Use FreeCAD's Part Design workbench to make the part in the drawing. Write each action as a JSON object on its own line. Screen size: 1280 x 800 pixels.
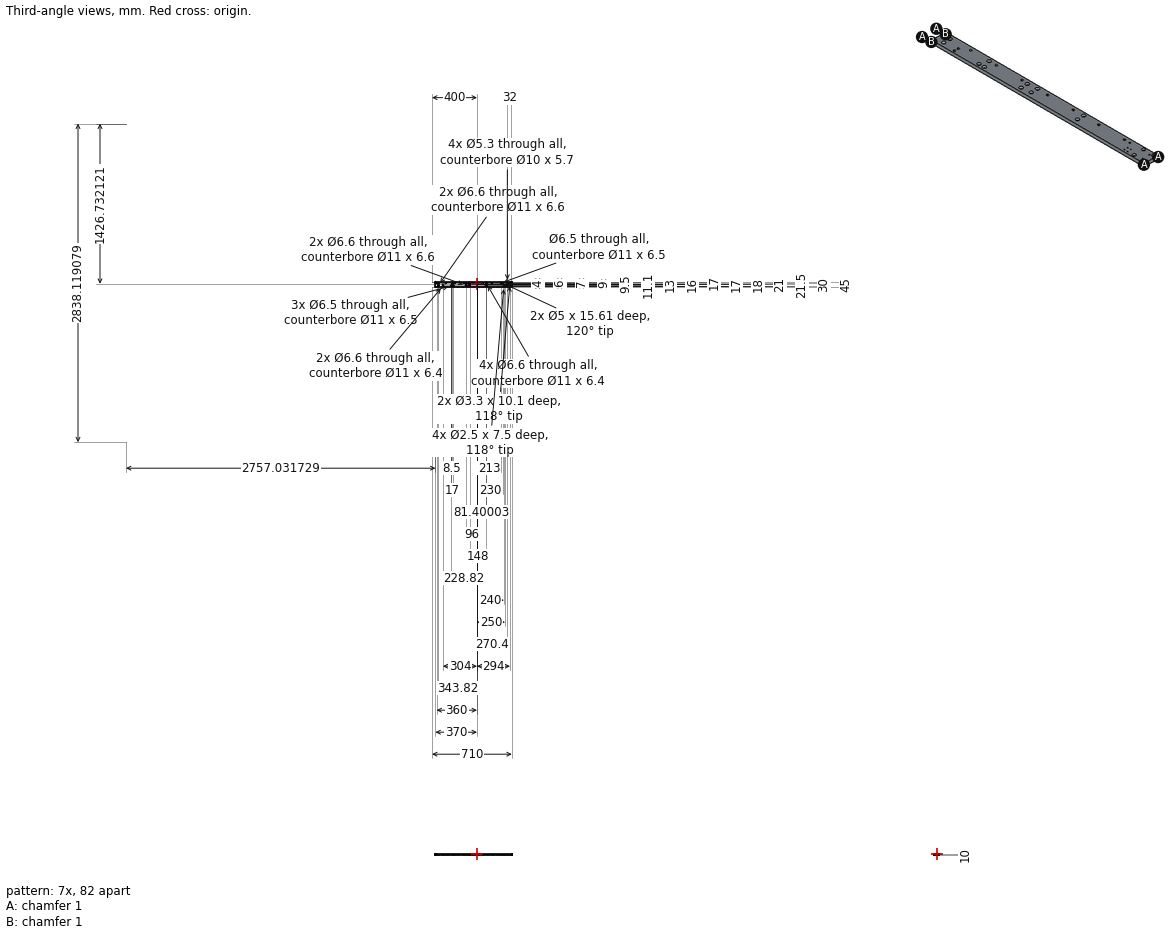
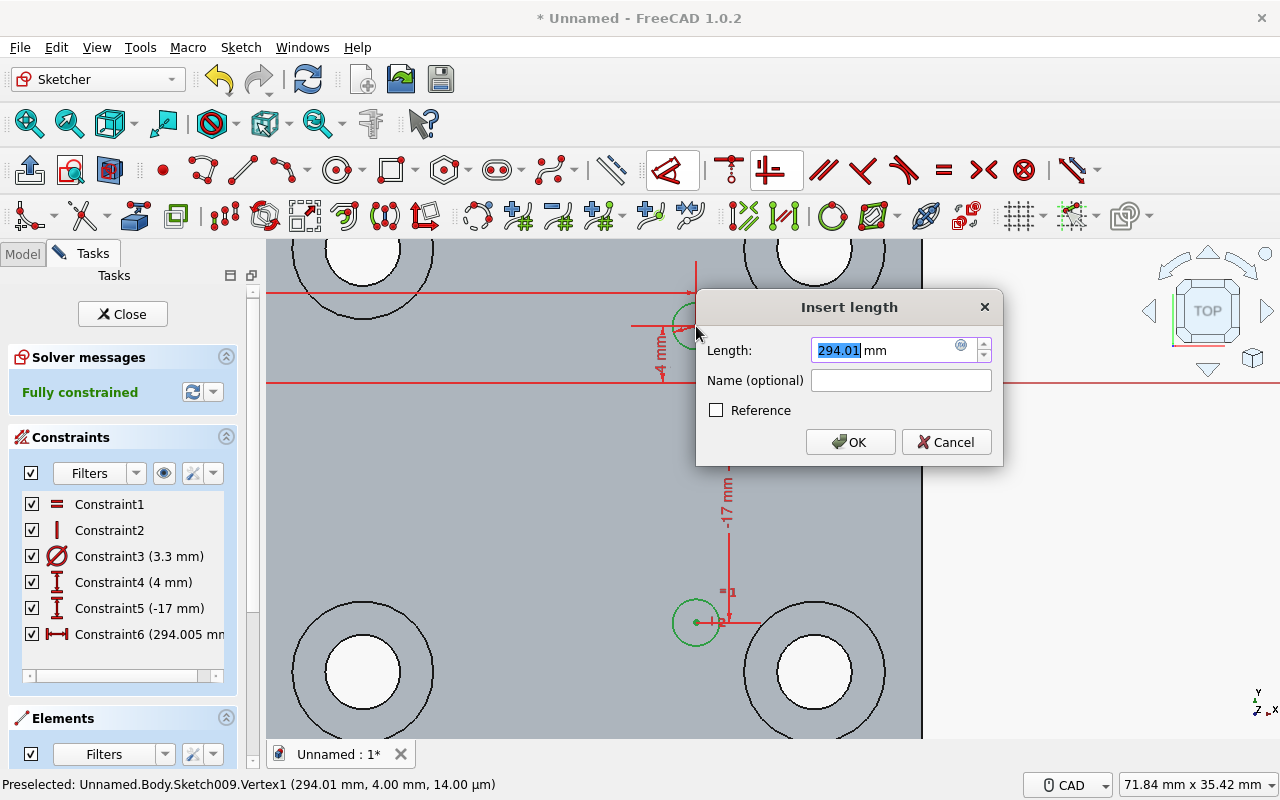
{"action": "type", "text": "294"}
{"action": "key", "text": "Return"}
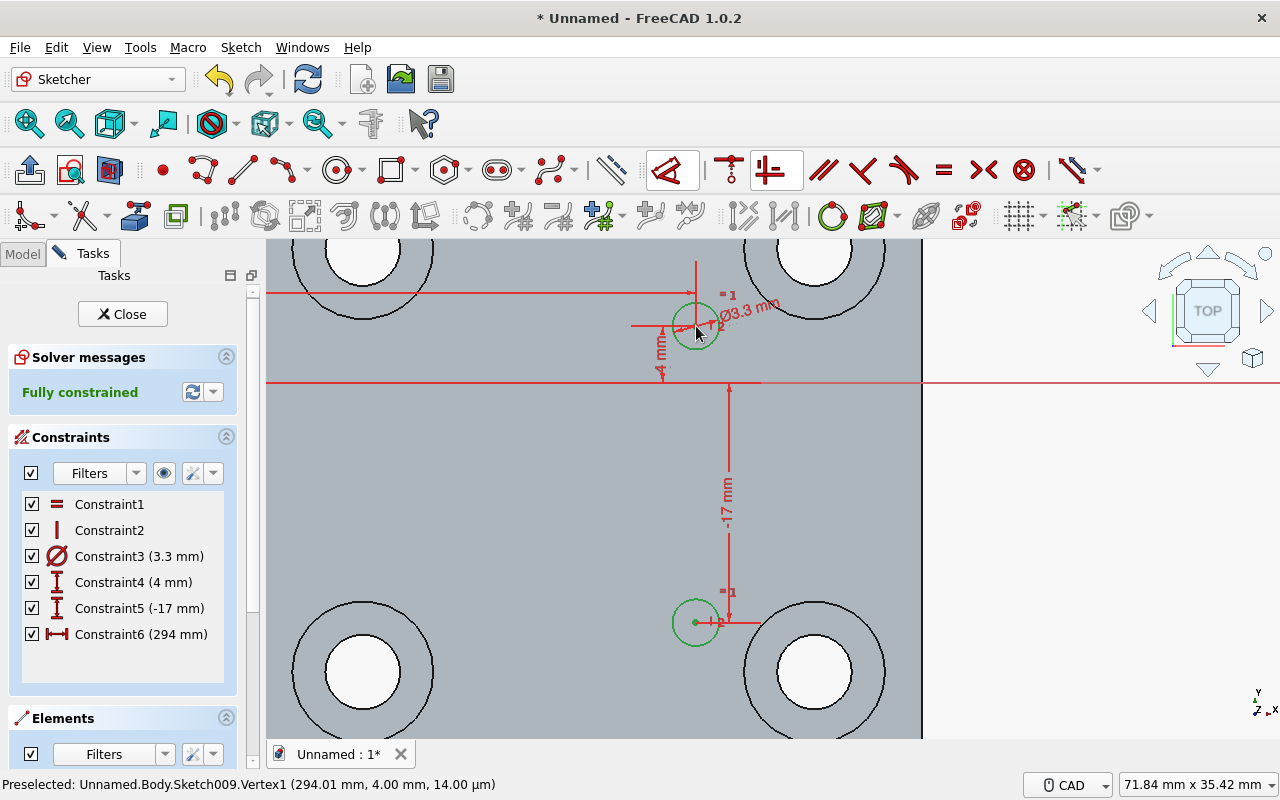
{"action": "left_click", "coordinate": [123, 314]}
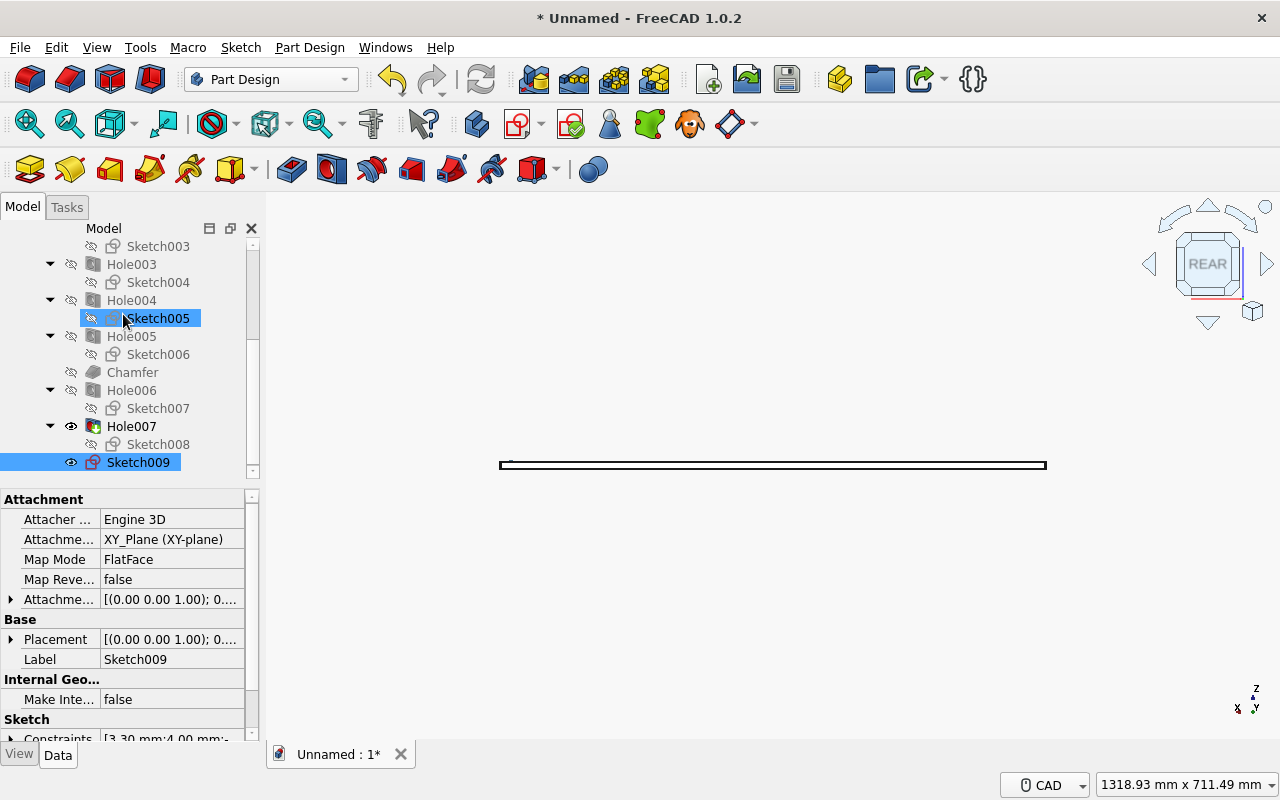
{"action": "left_click", "coordinate": [332, 170]}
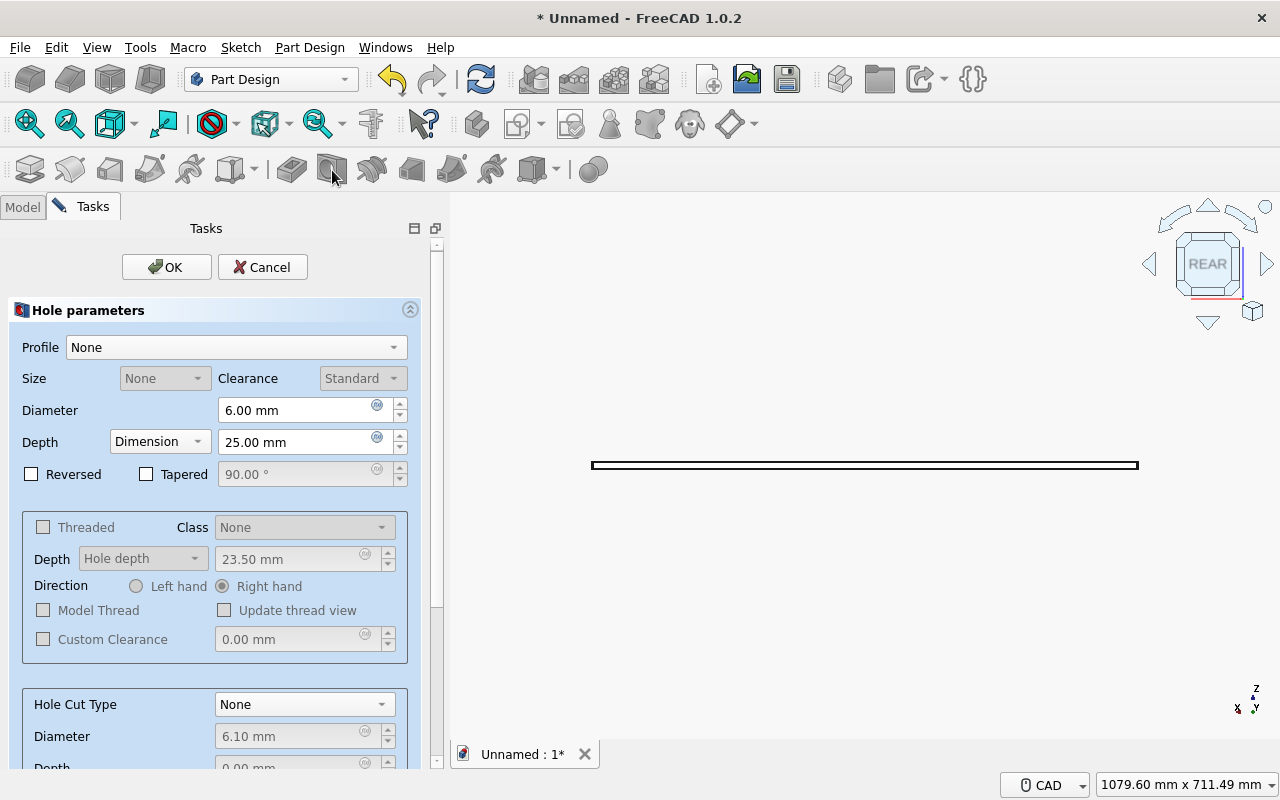
{"action": "triple_click", "coordinate": [305, 410]}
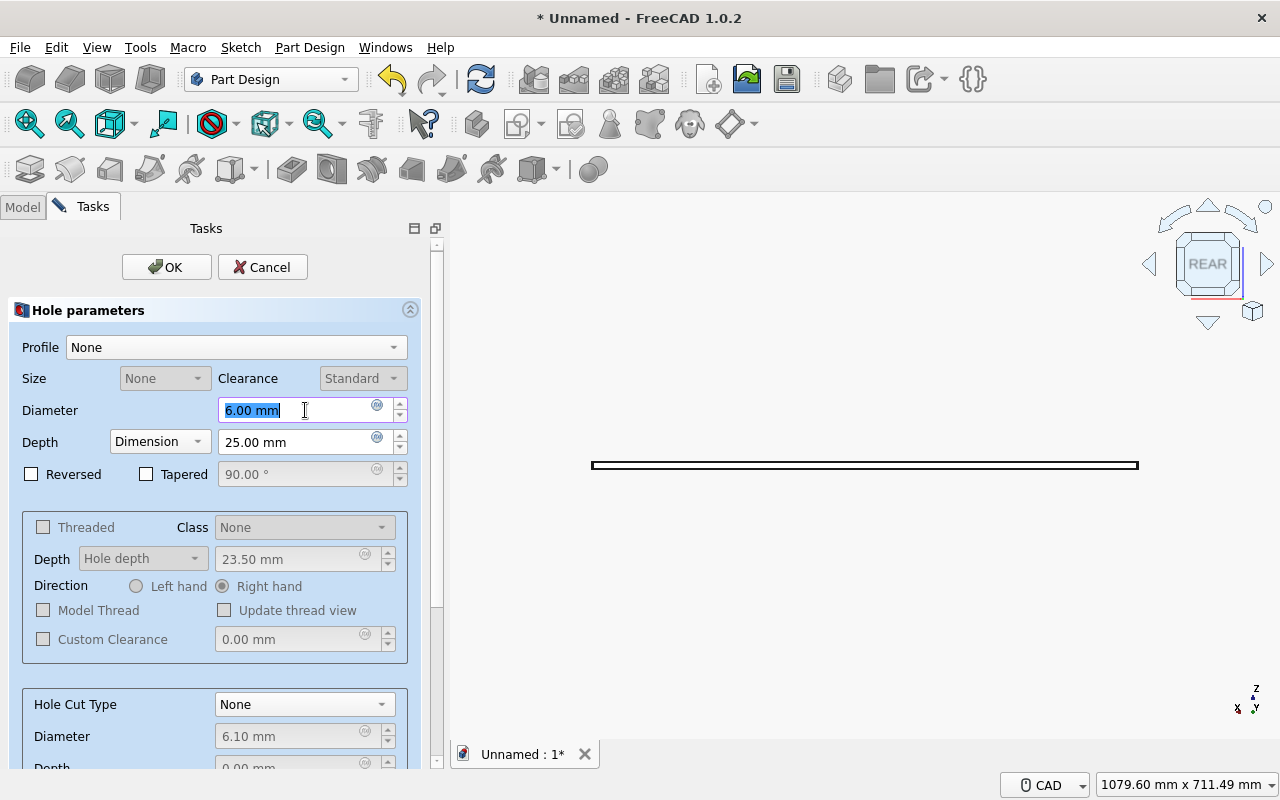
{"action": "type", "text": "3.3"}
{"action": "key", "text": "Tab"}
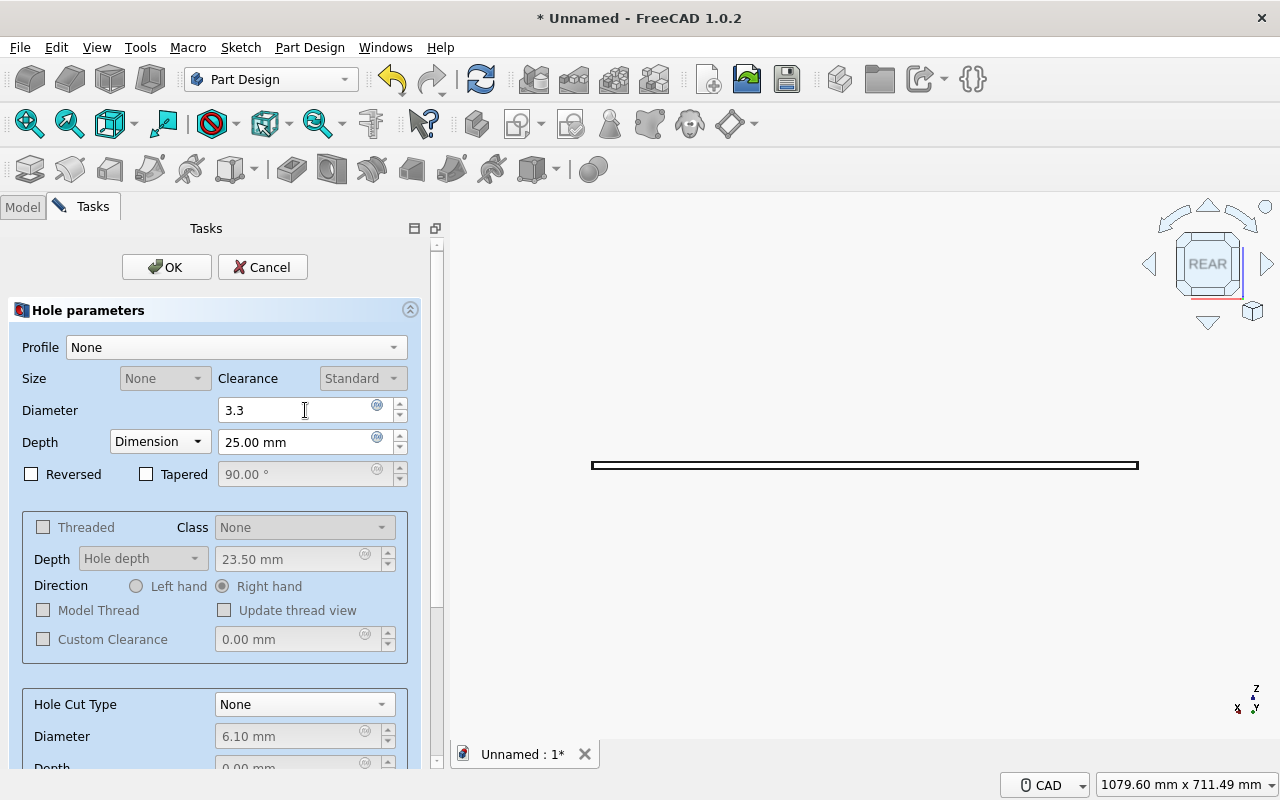
{"action": "triple_click", "coordinate": [305, 442]}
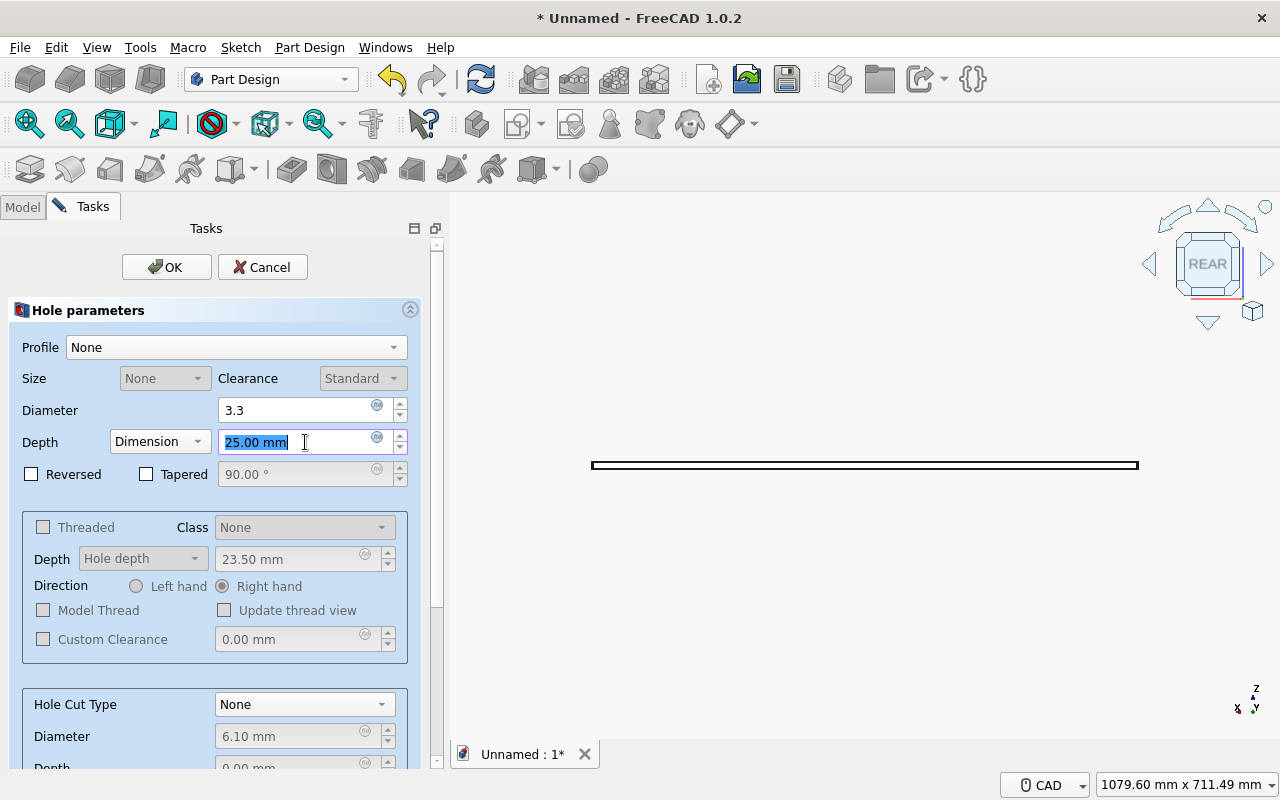
{"action": "type", "text": "10.1"}
{"action": "key", "text": "Tab"}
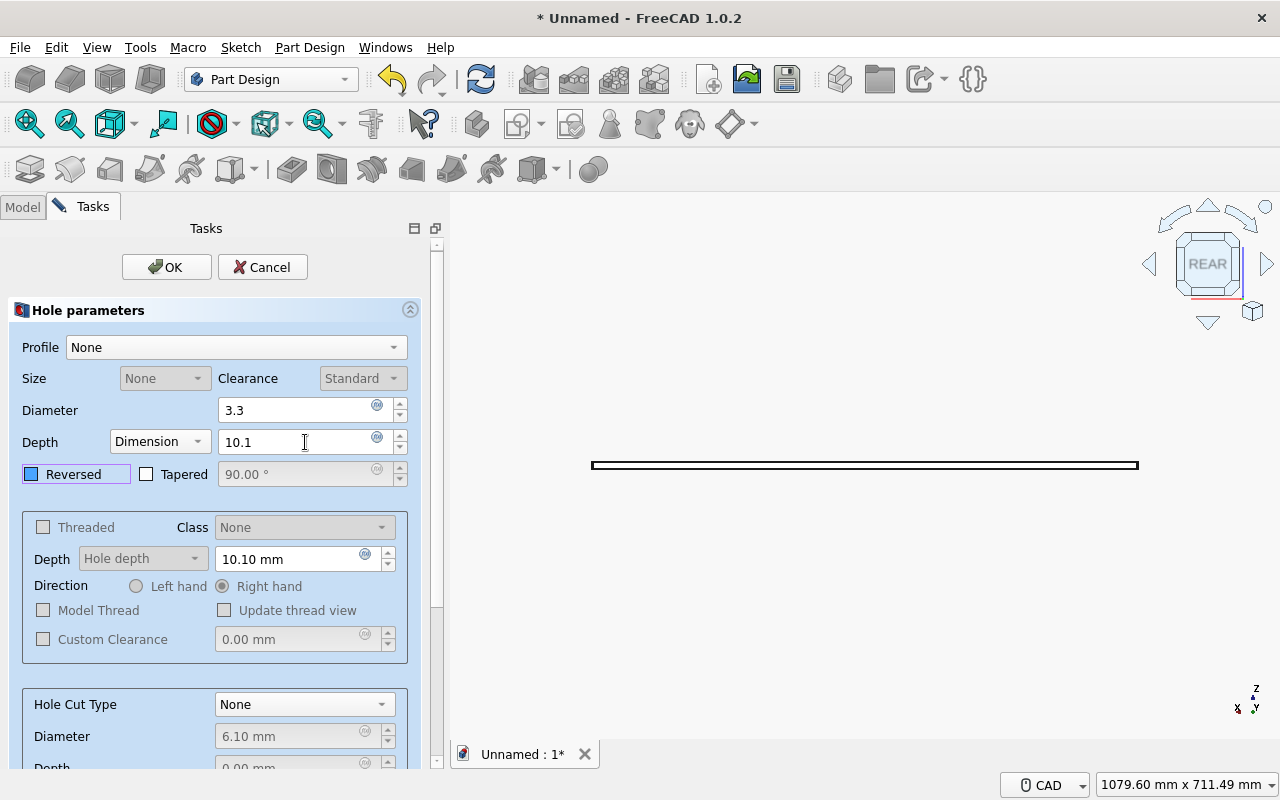
{"action": "left_click", "coordinate": [167, 267]}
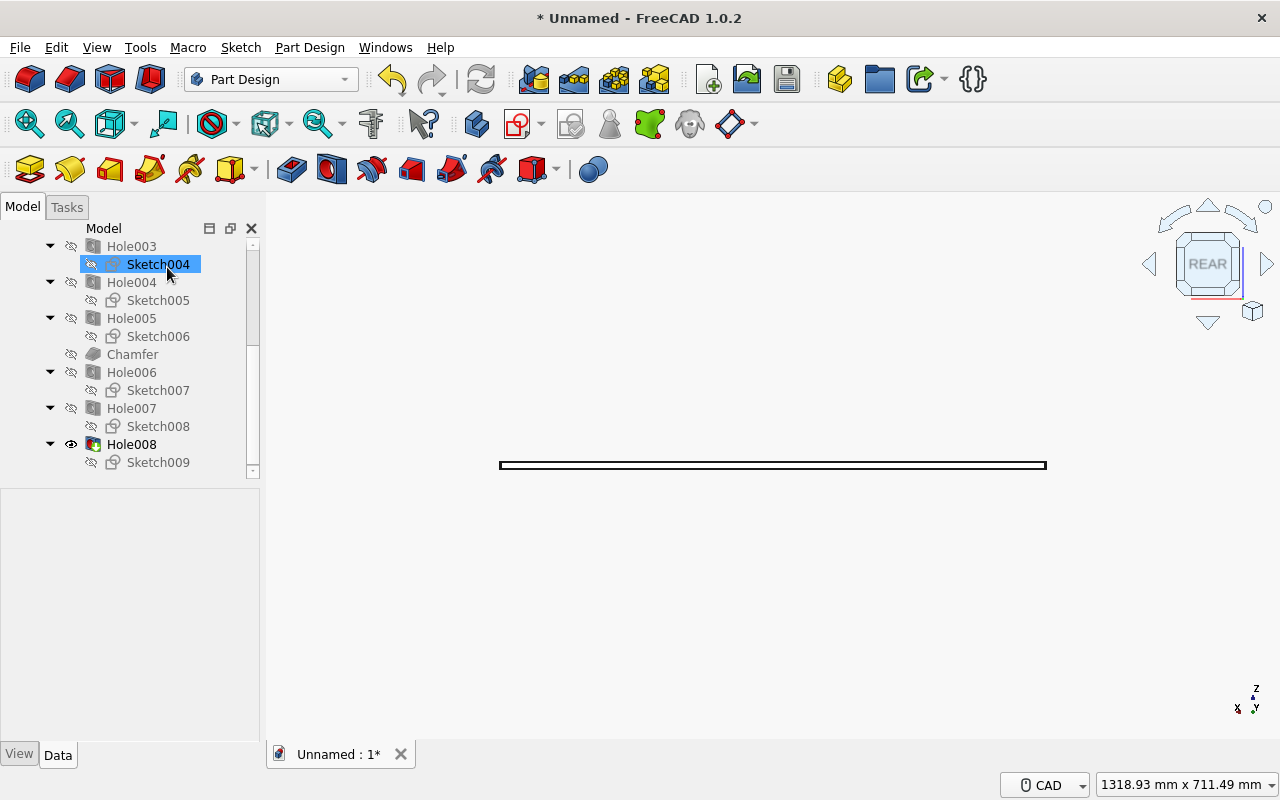
{"action": "key", "text": "0"}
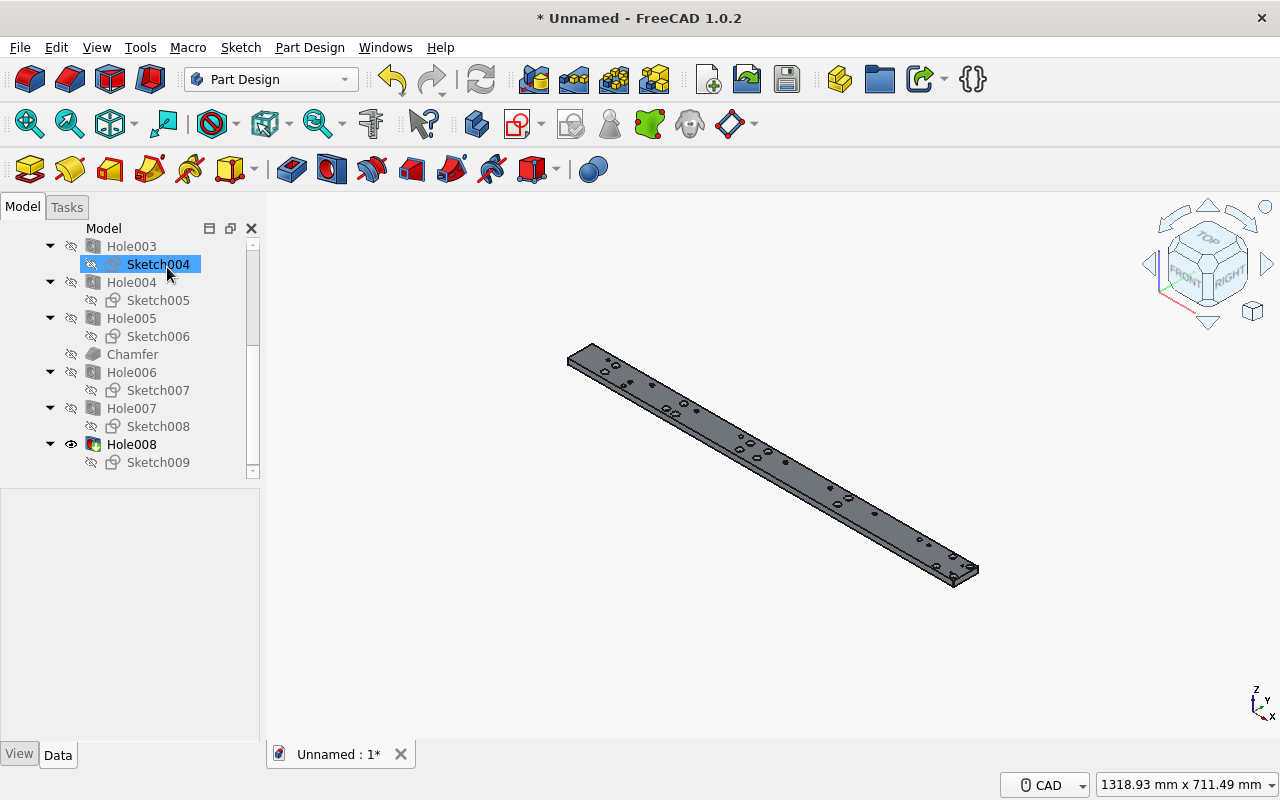
{"action": "left_click", "coordinate": [30, 124]}